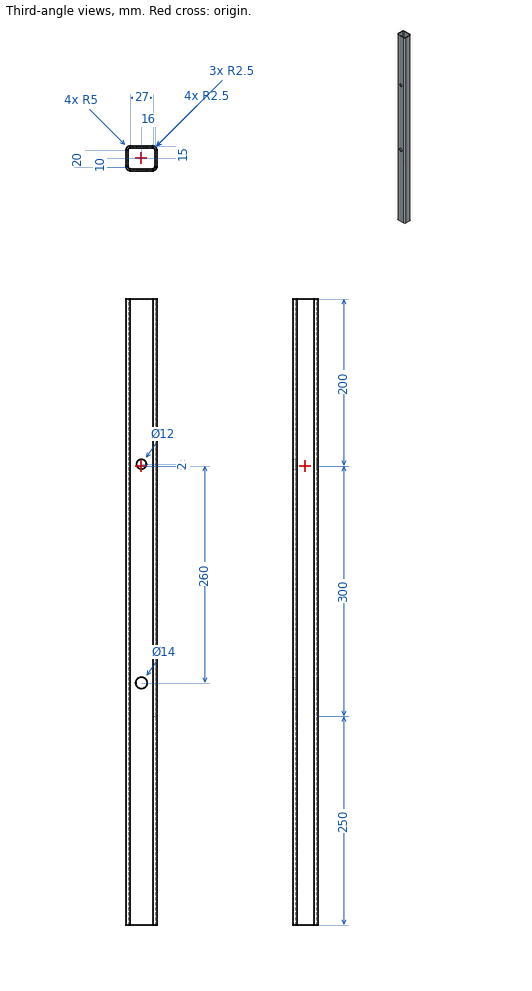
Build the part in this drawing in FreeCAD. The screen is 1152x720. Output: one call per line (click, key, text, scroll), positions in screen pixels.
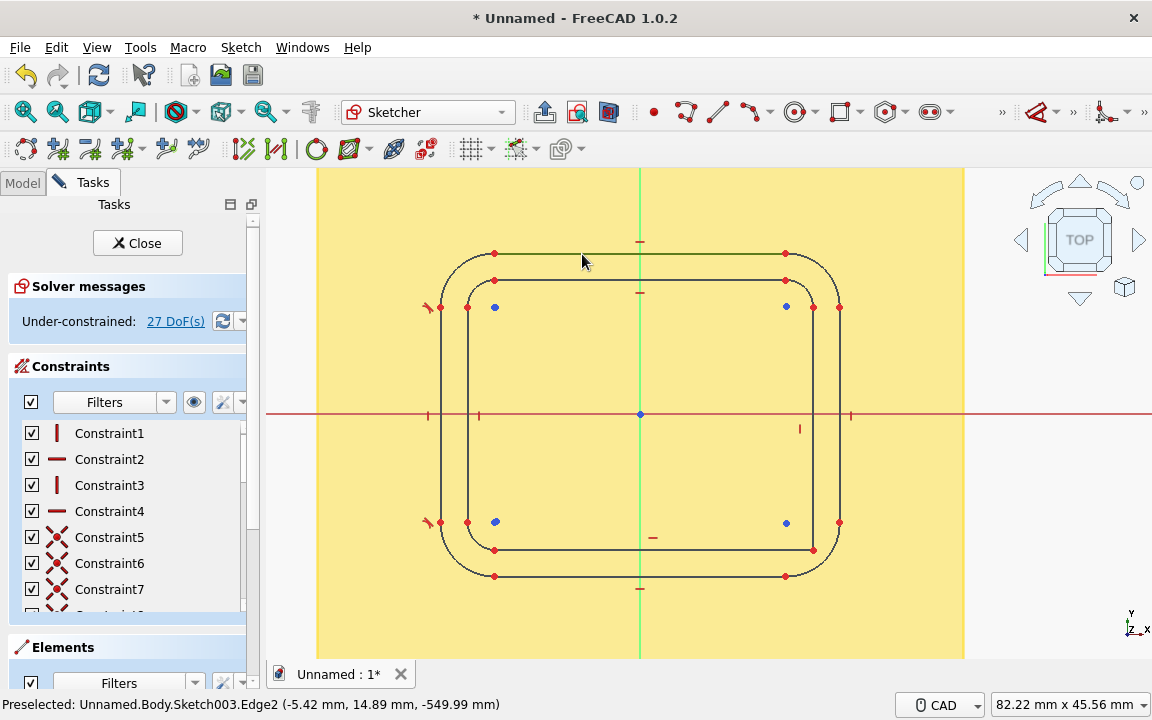
click(470, 259)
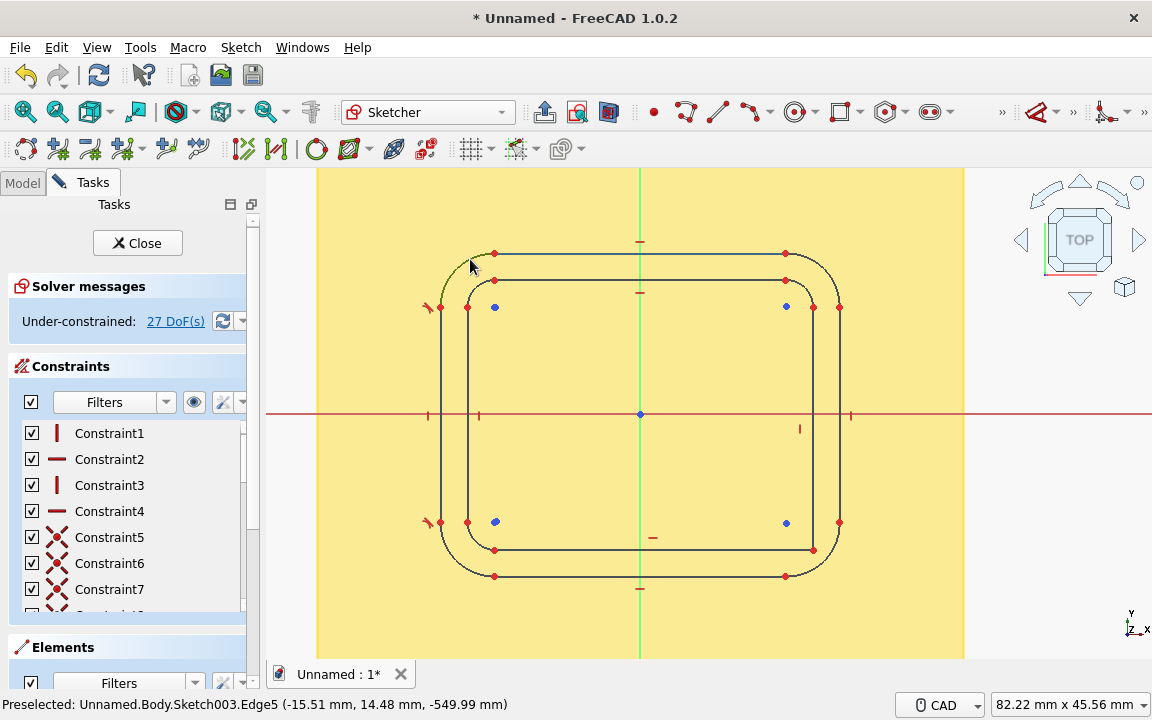
key(t)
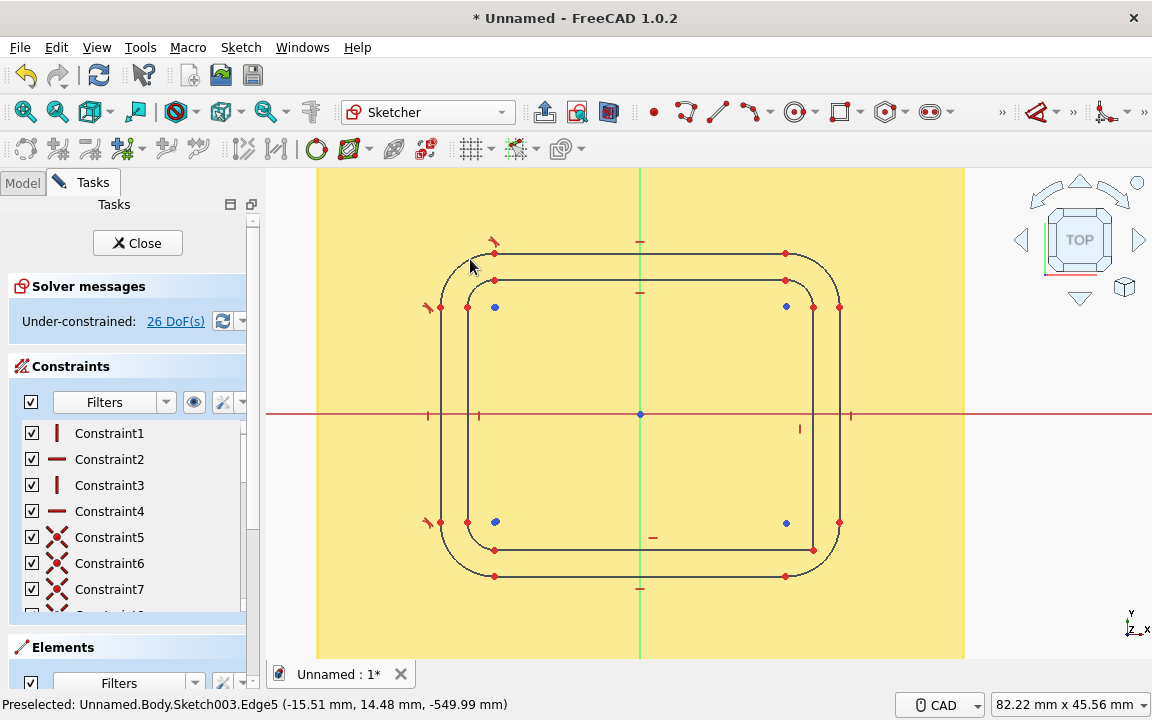
click(582, 254)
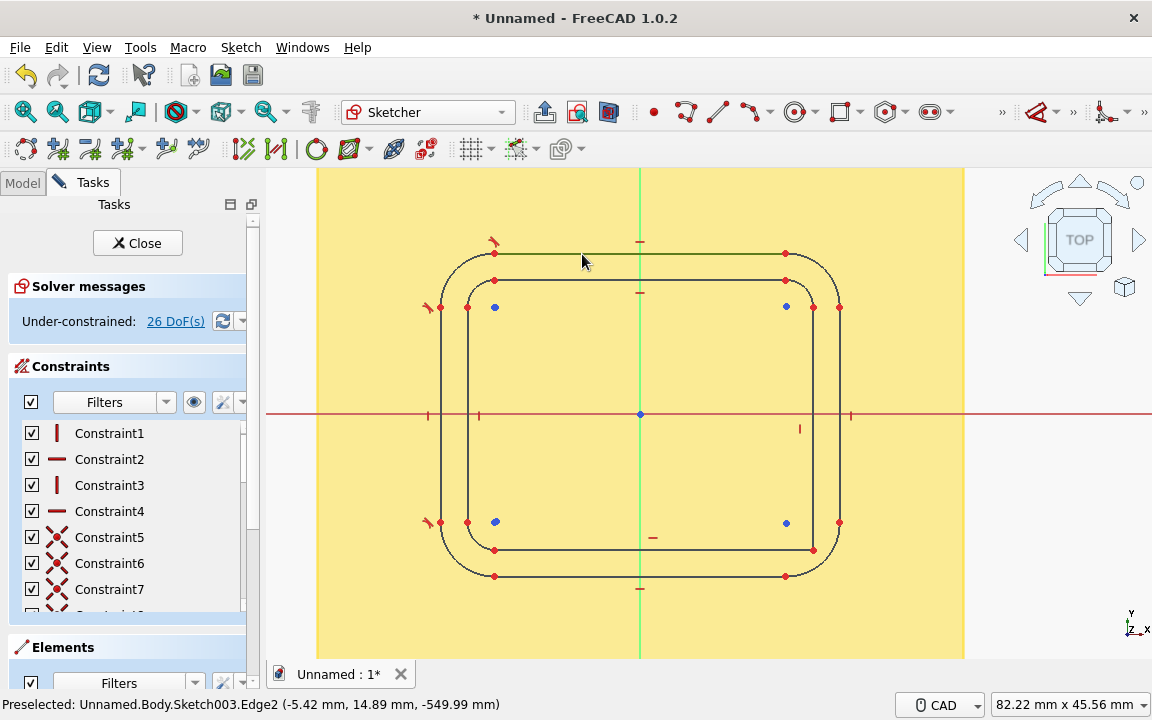
click(834, 283)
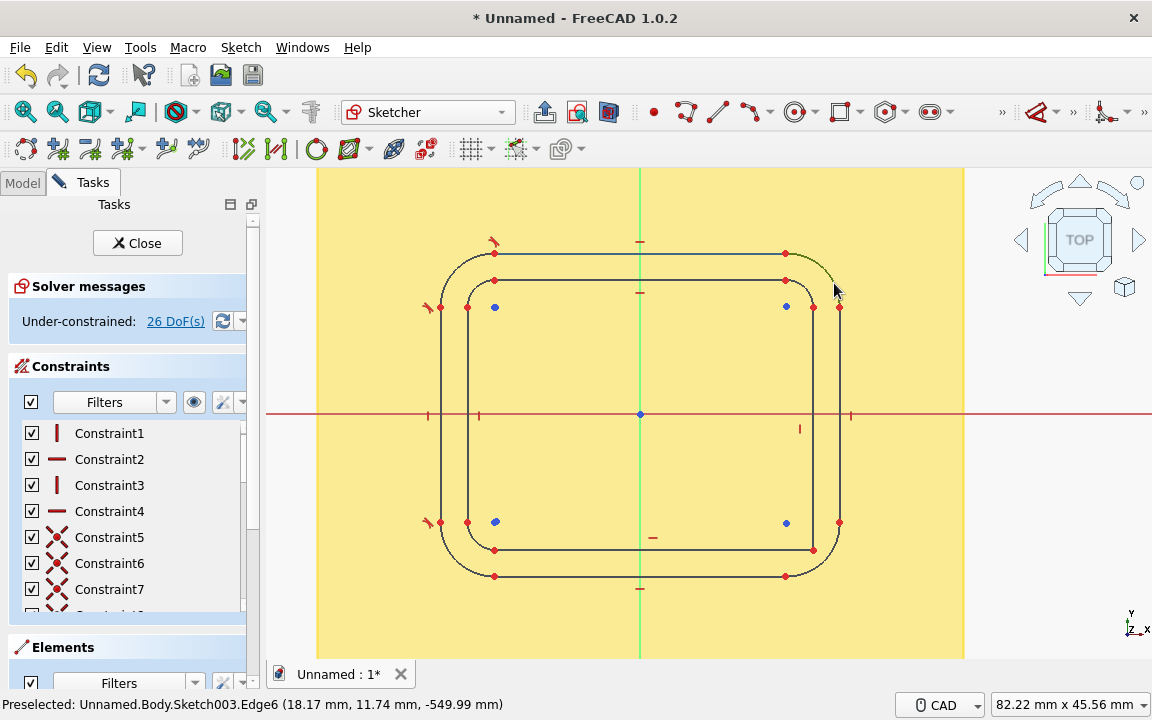
key(t)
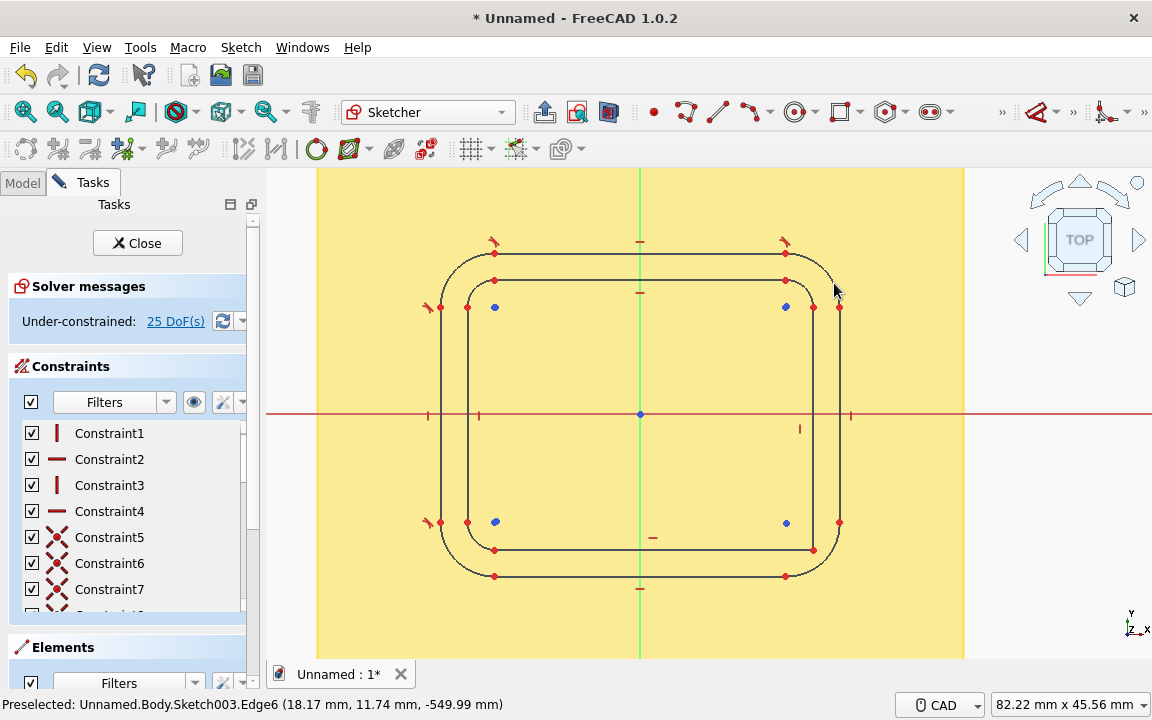
click(840, 372)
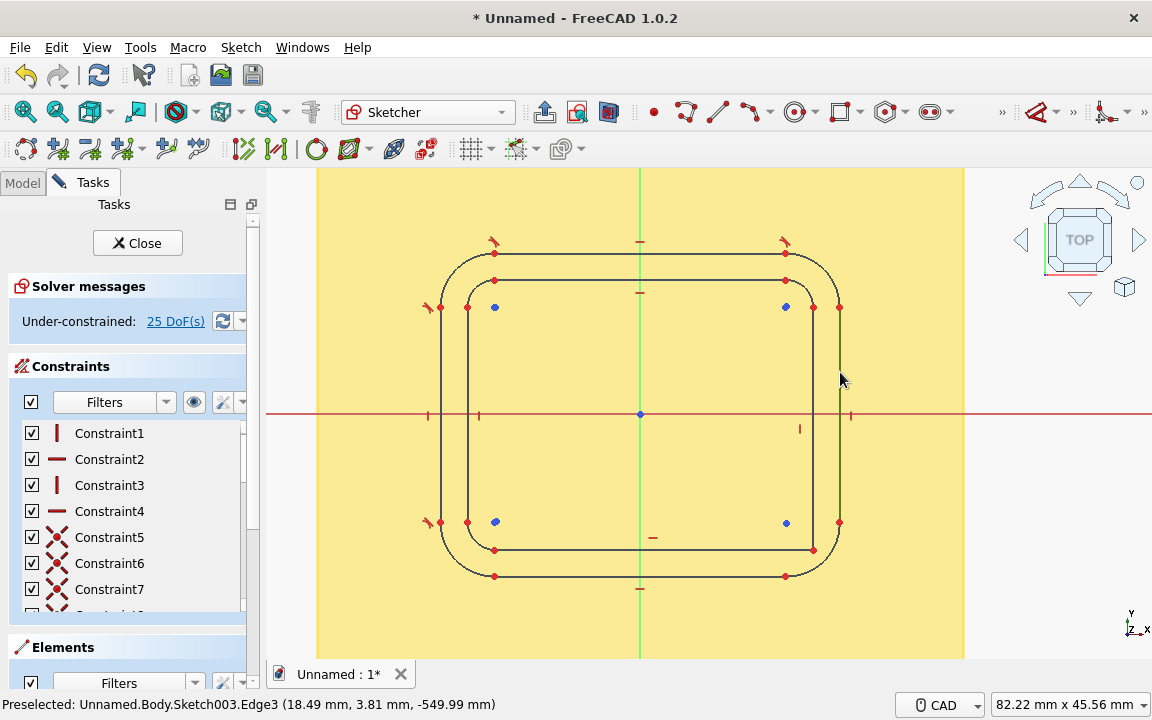
click(834, 283)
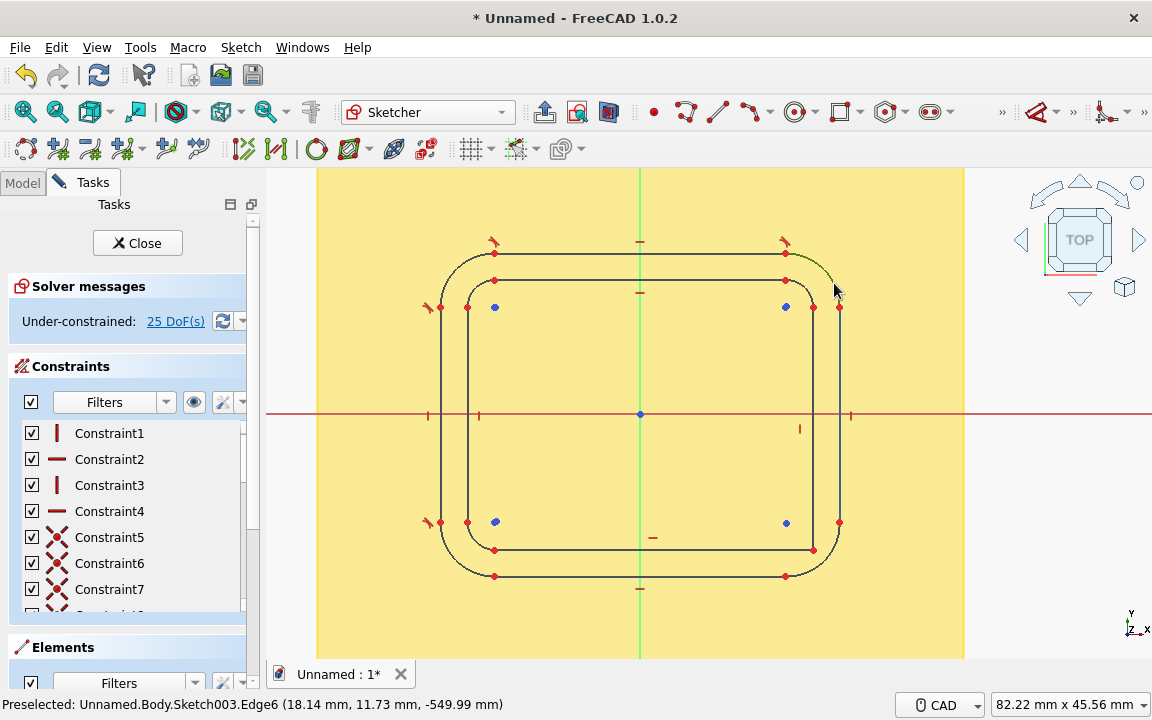
key(t)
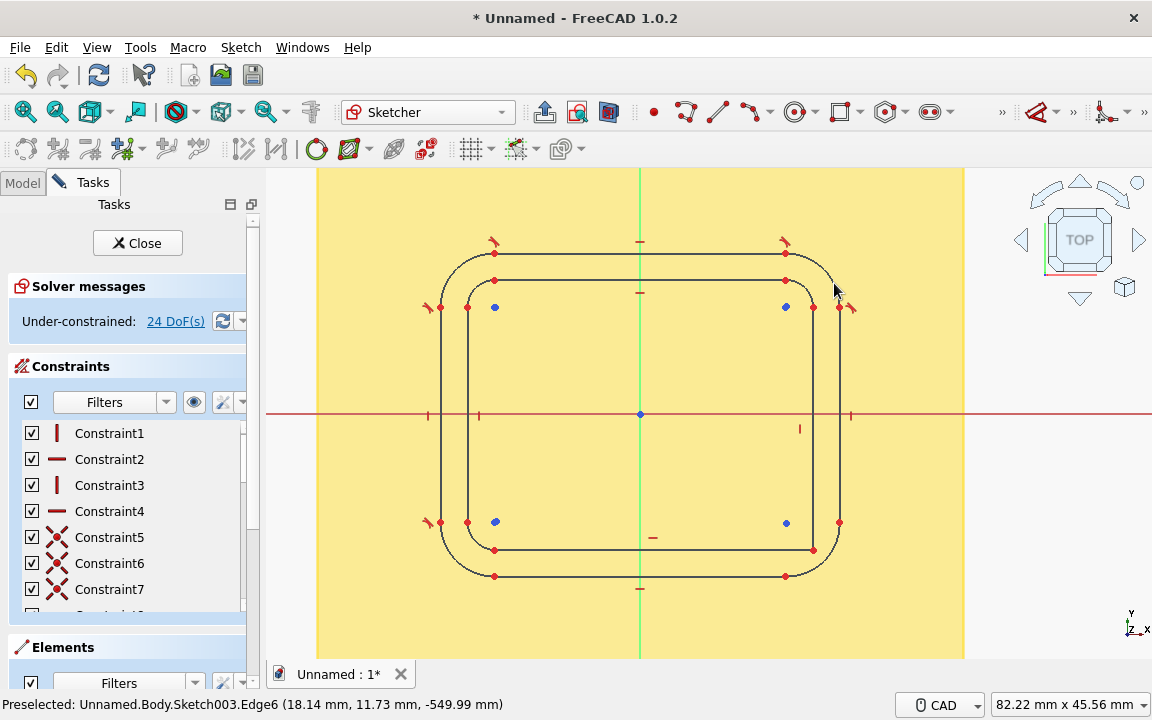
click(840, 372)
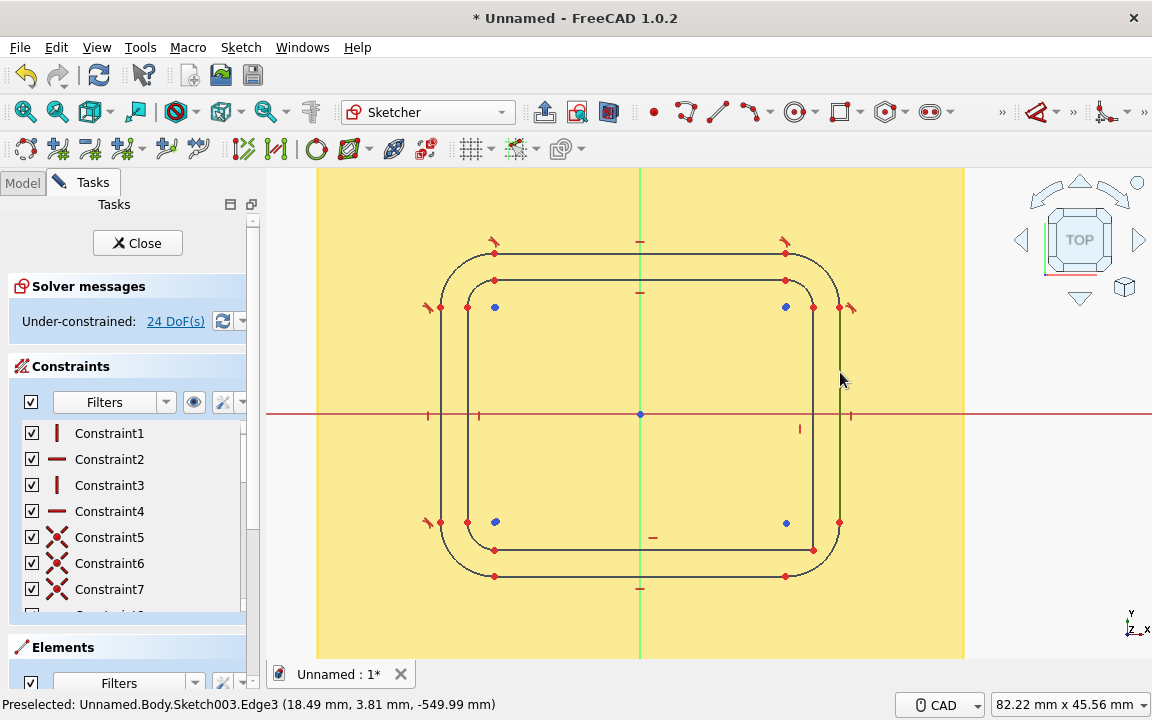
click(810, 571)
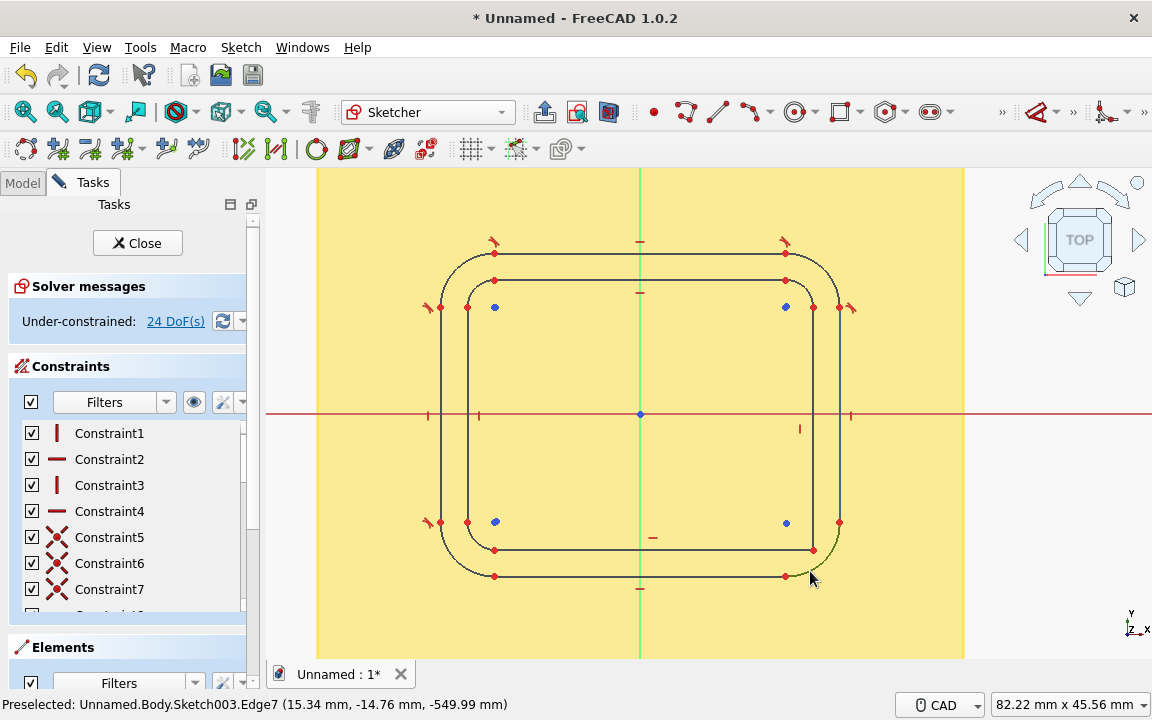
key(t)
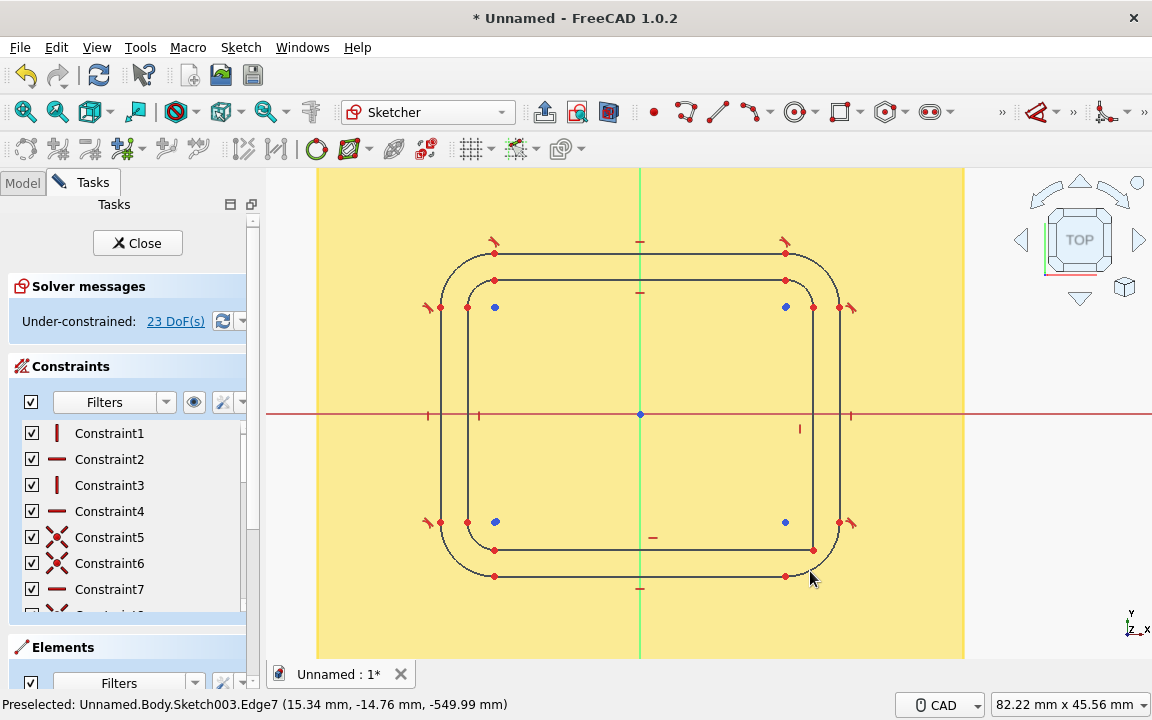
click(698, 577)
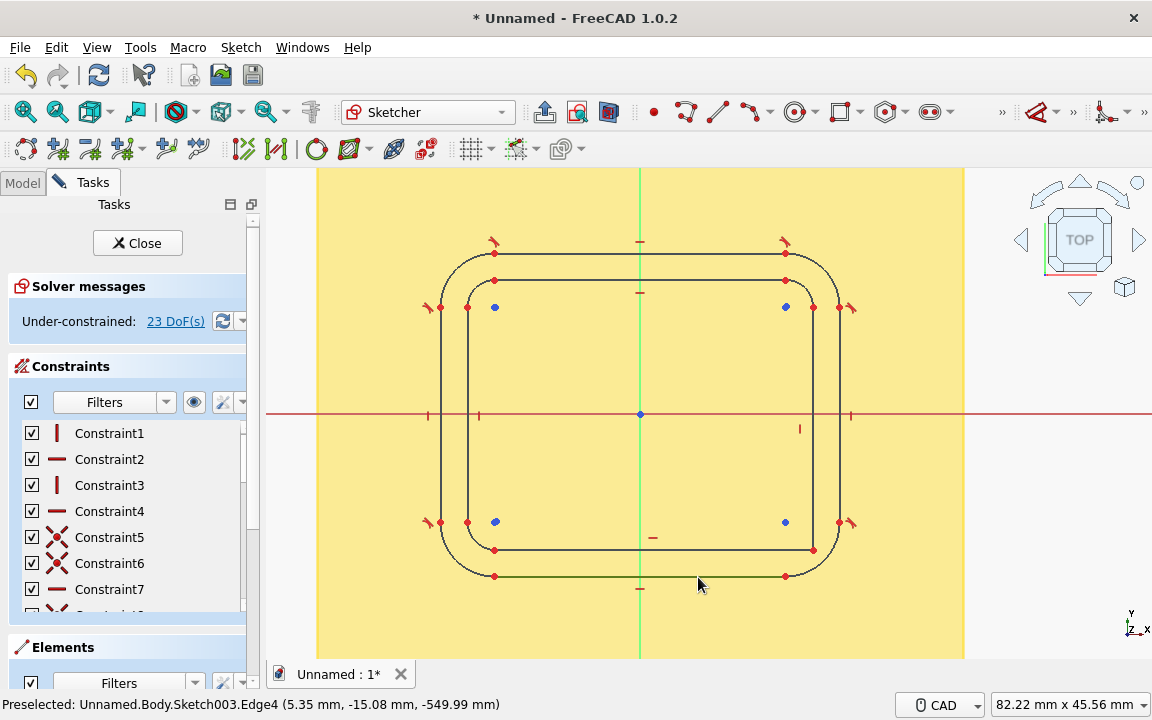
click(810, 571)